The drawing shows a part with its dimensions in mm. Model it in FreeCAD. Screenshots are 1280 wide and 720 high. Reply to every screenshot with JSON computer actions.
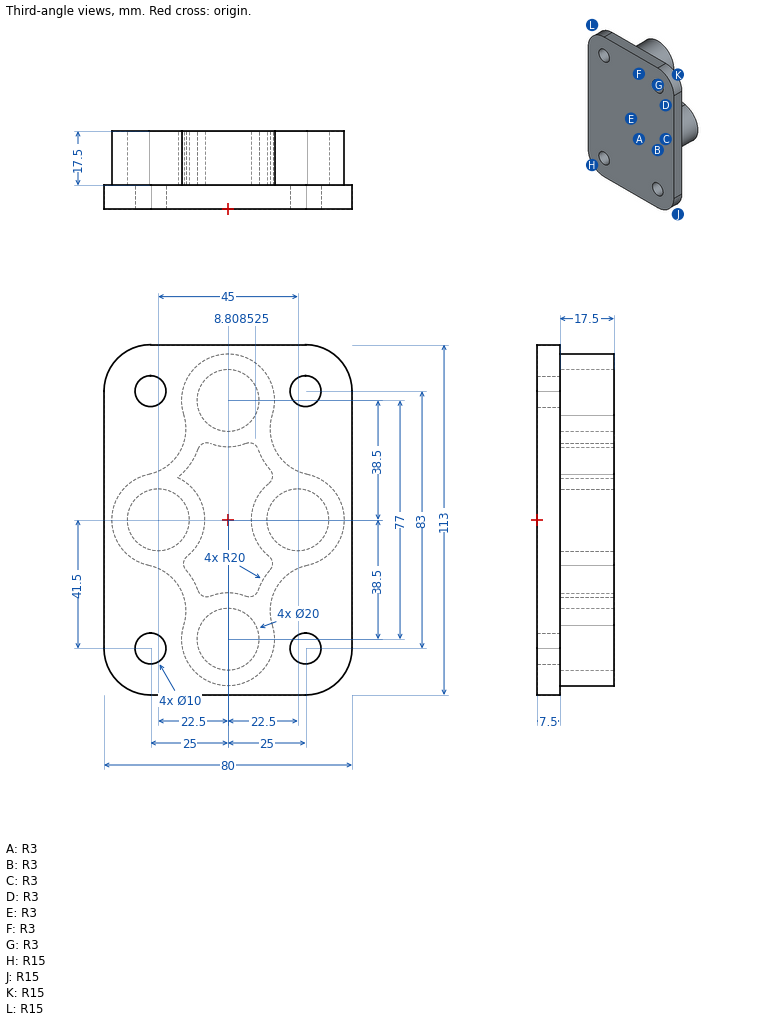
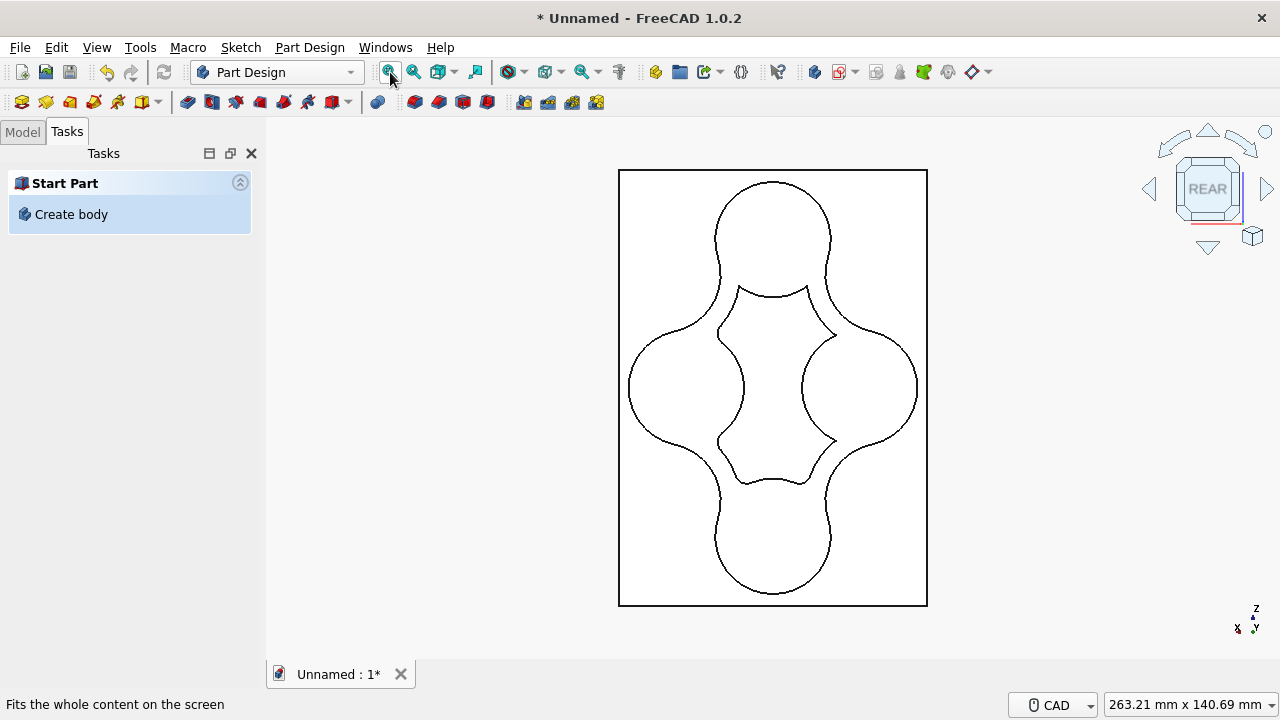
{"action": "key", "text": "6"}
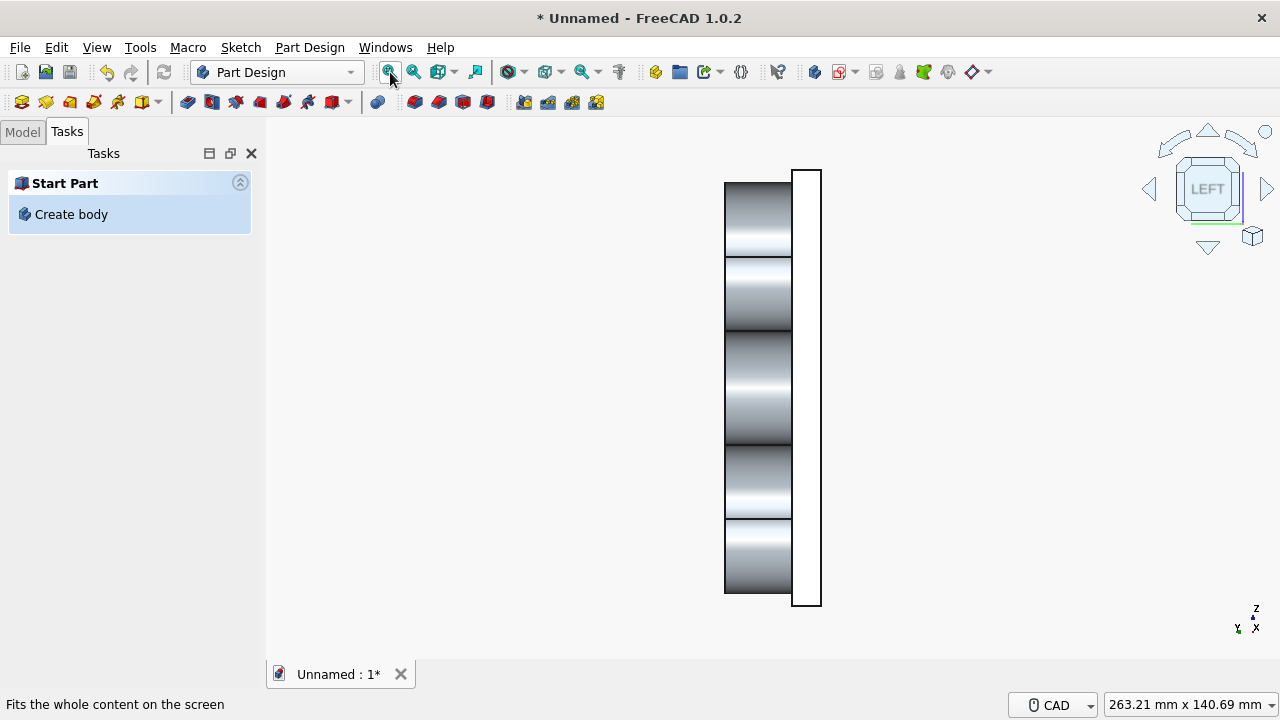
{"action": "key", "text": "v 3"}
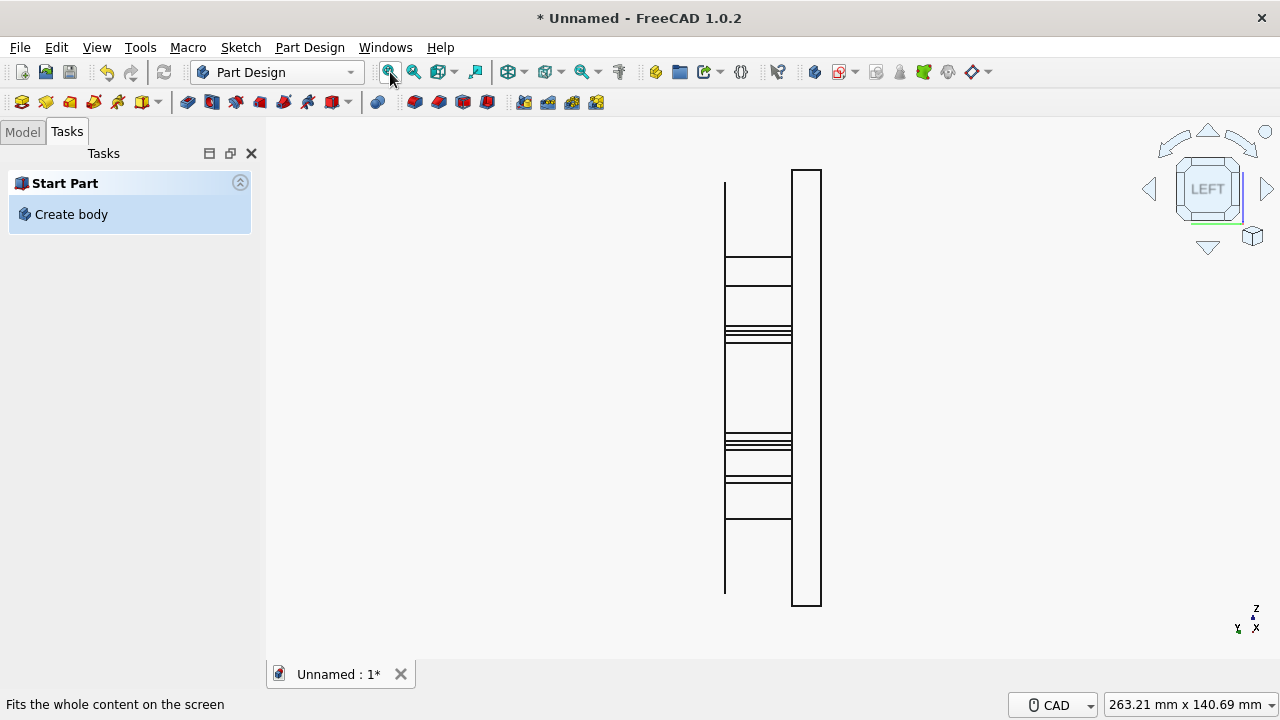
{"action": "key", "text": "0"}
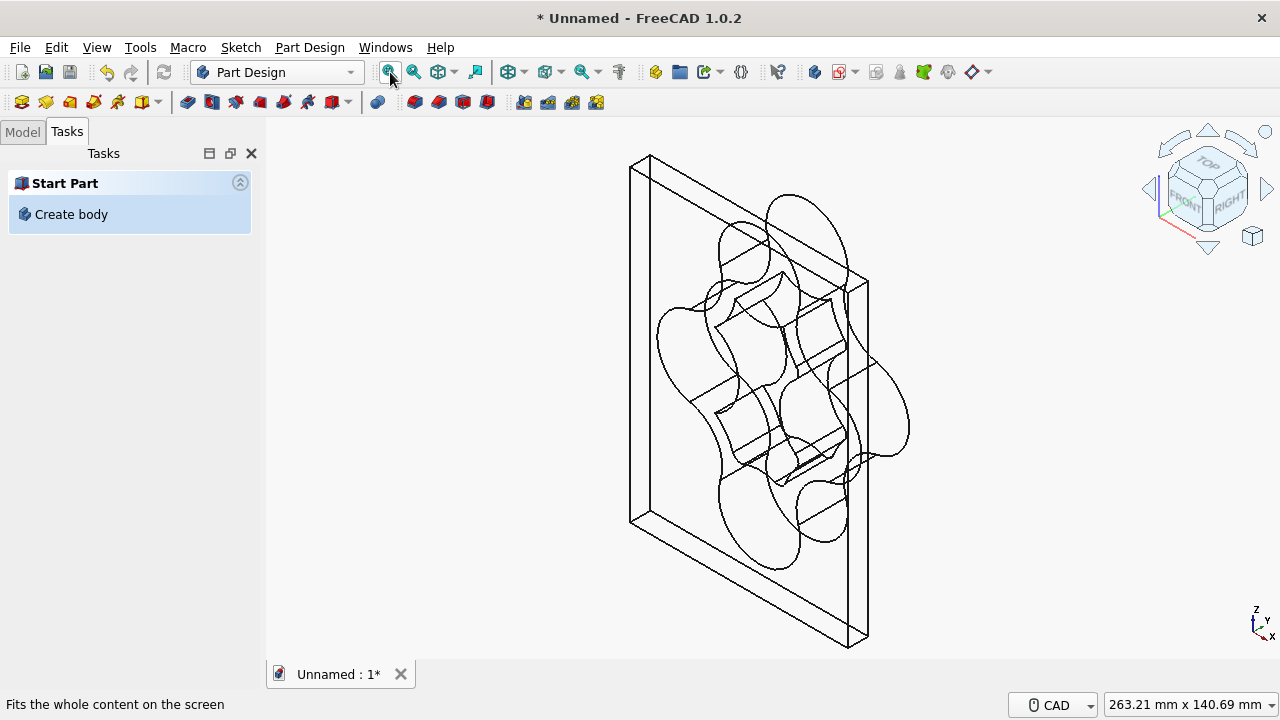
{"action": "left_click", "coordinate": [744, 396]}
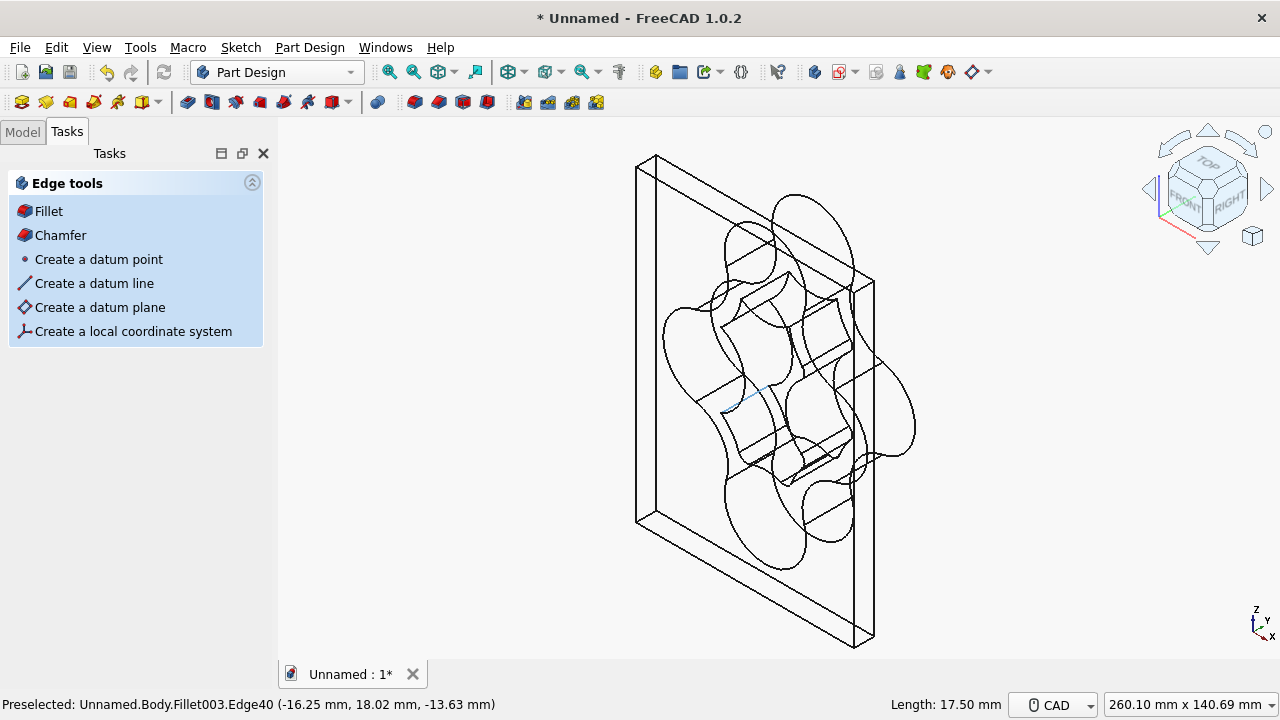
{"action": "key", "text": "v 1"}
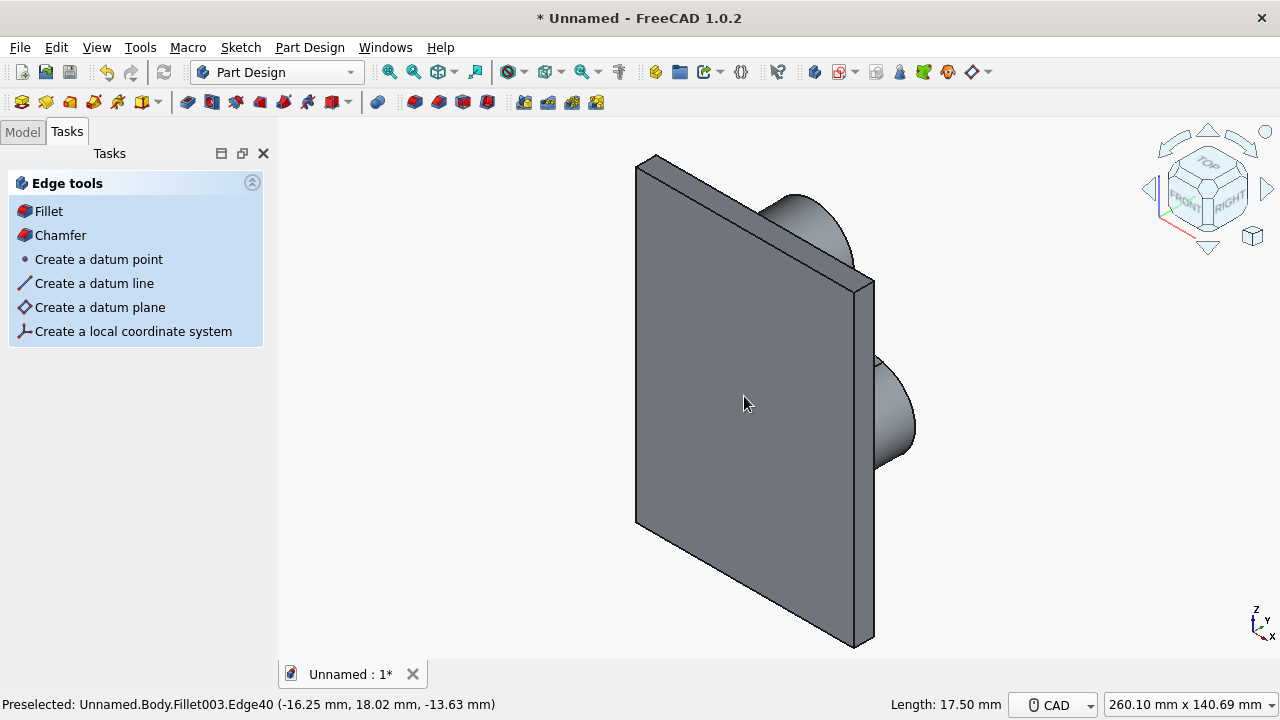
{"action": "left_click", "coordinate": [416, 102]}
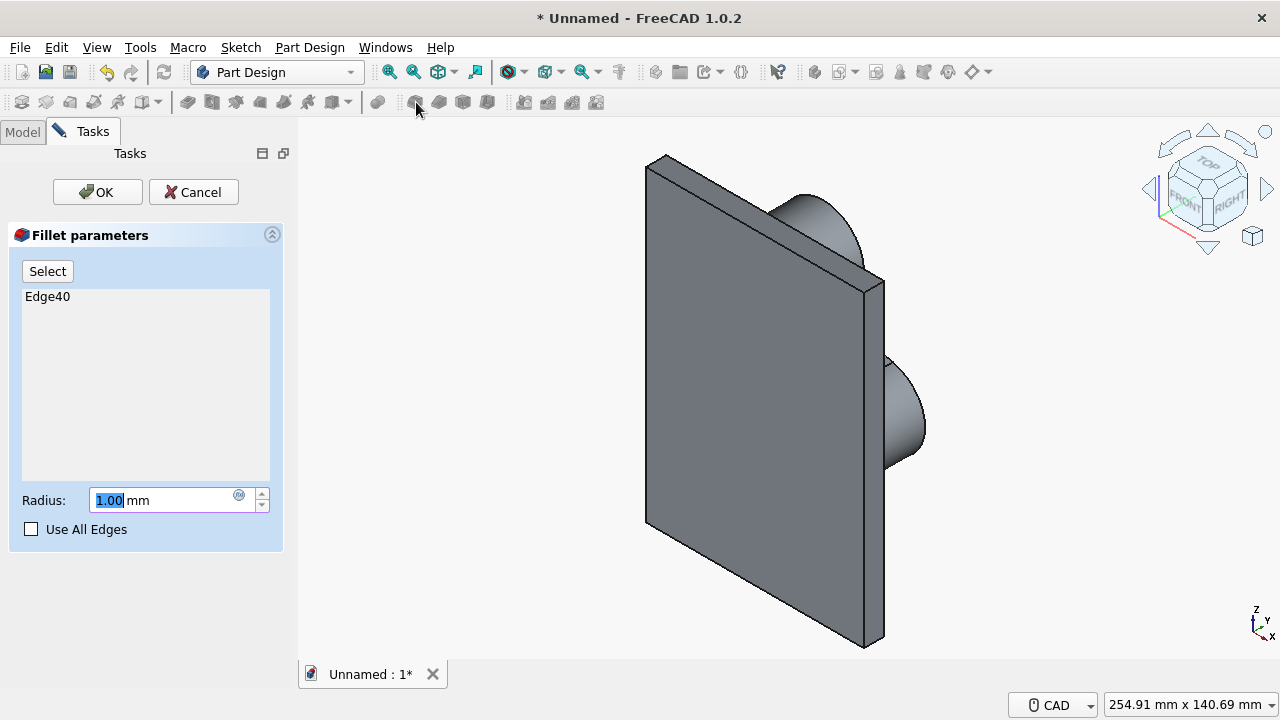
{"action": "type", "text": "3"}
{"action": "key", "text": "Tab"}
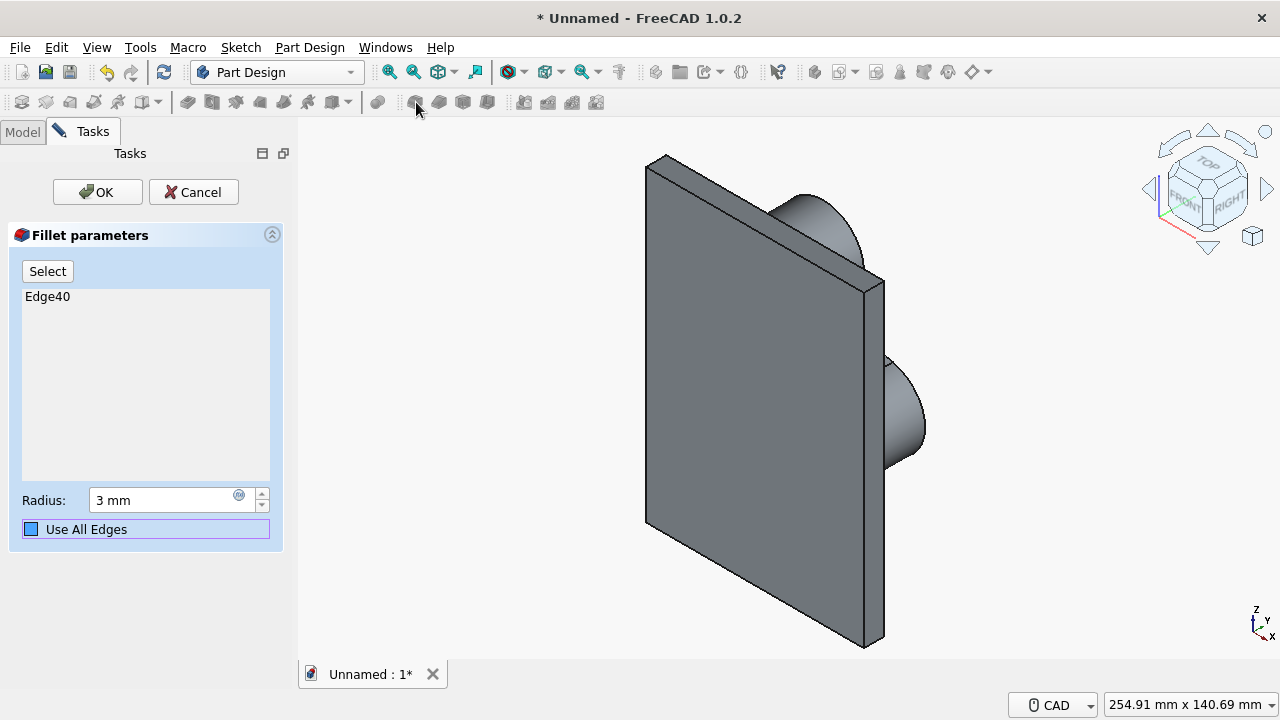
{"action": "left_click", "coordinate": [98, 192]}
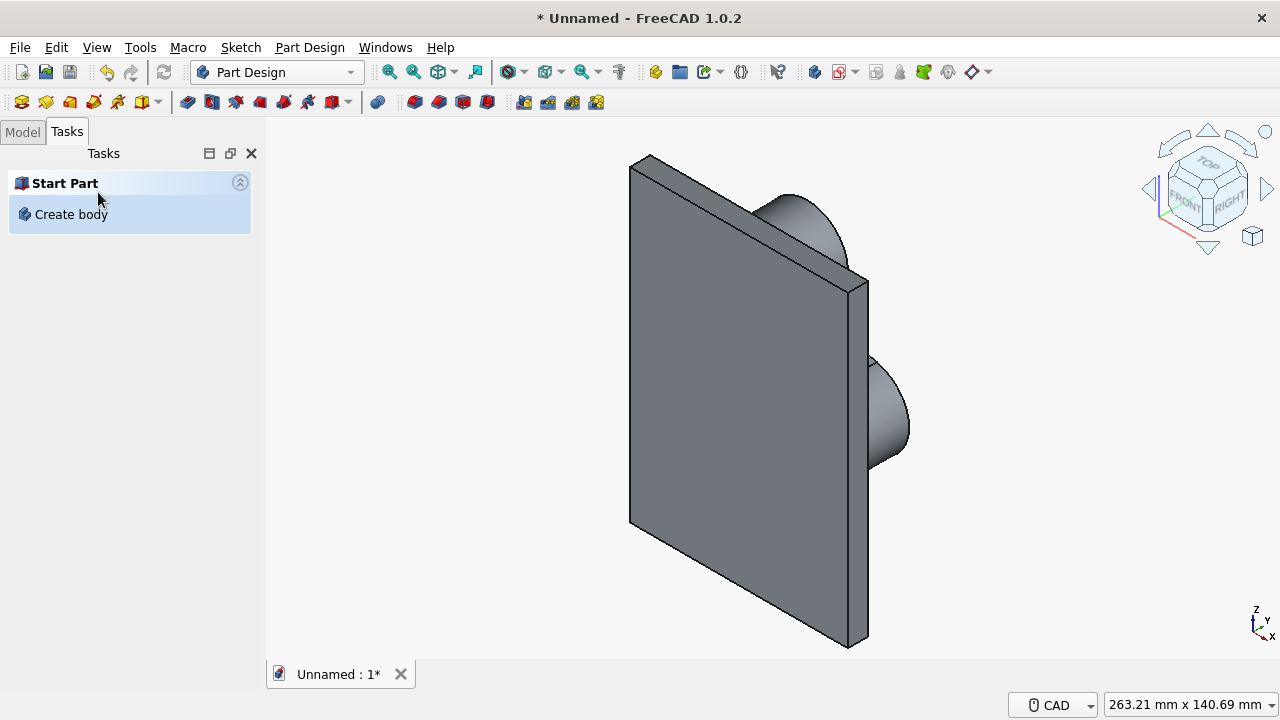
{"action": "key", "text": "2"}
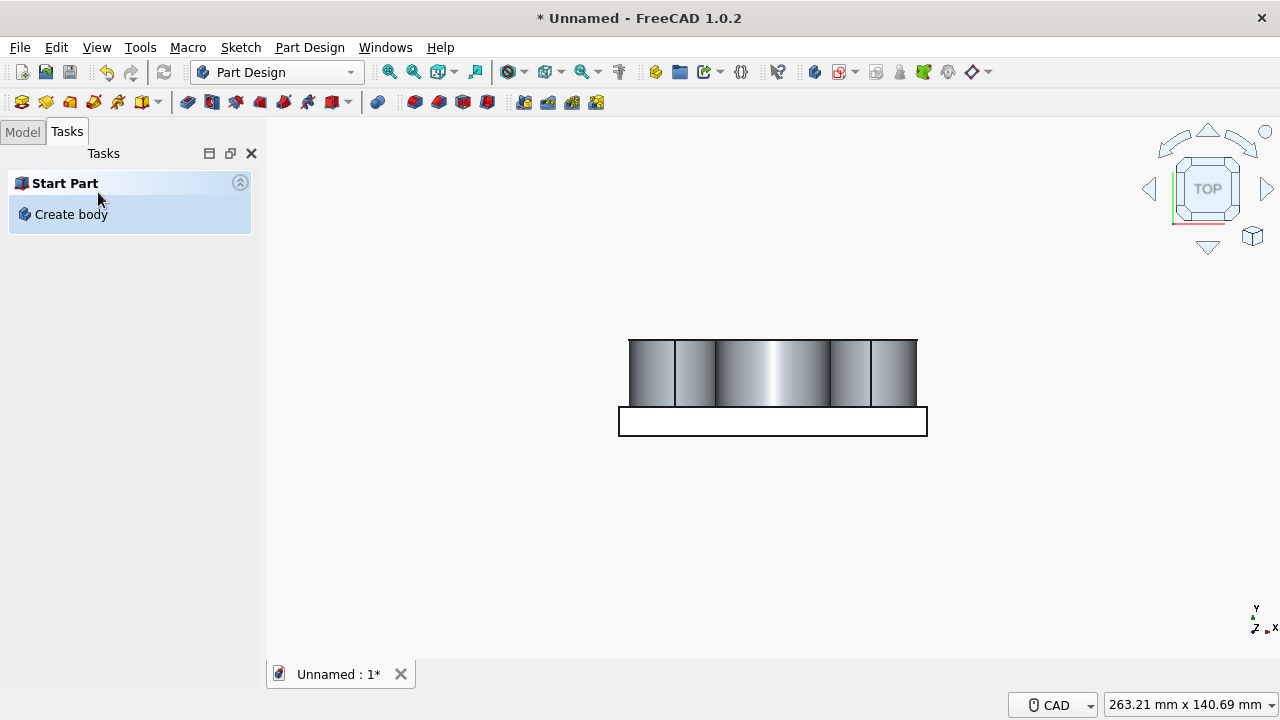
{"action": "key", "text": "v f"}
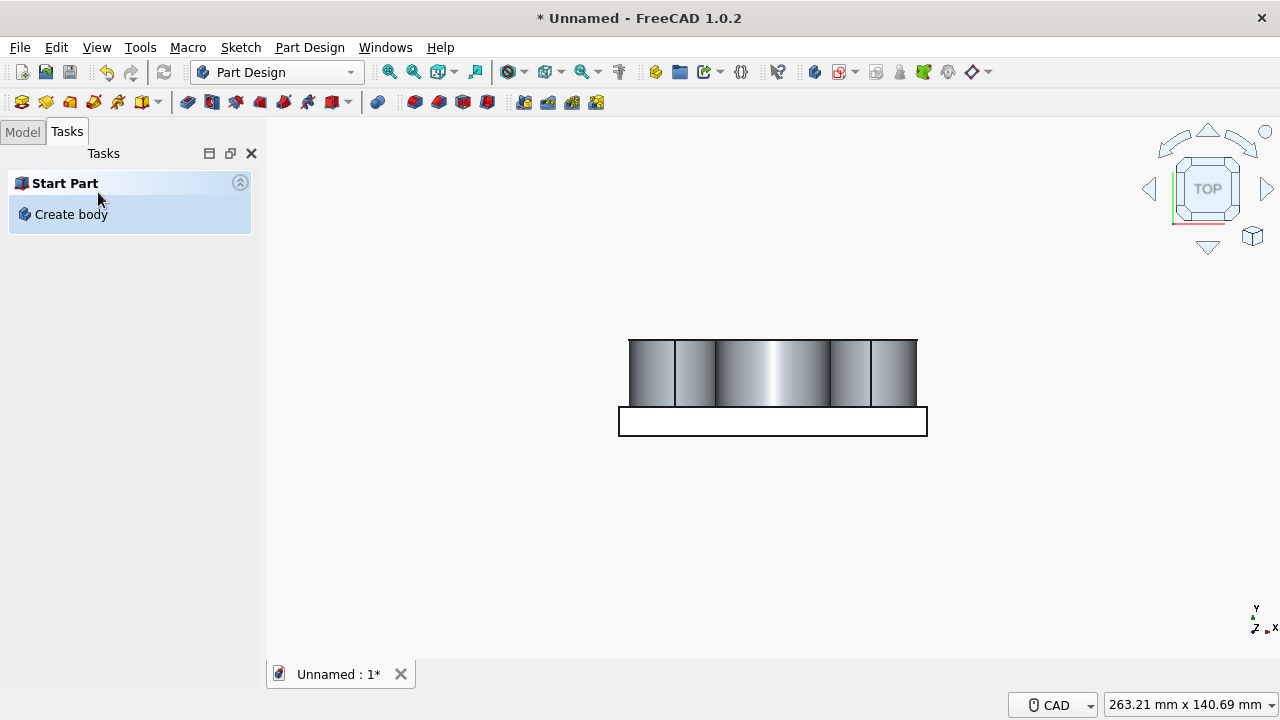
{"action": "key", "text": "0"}